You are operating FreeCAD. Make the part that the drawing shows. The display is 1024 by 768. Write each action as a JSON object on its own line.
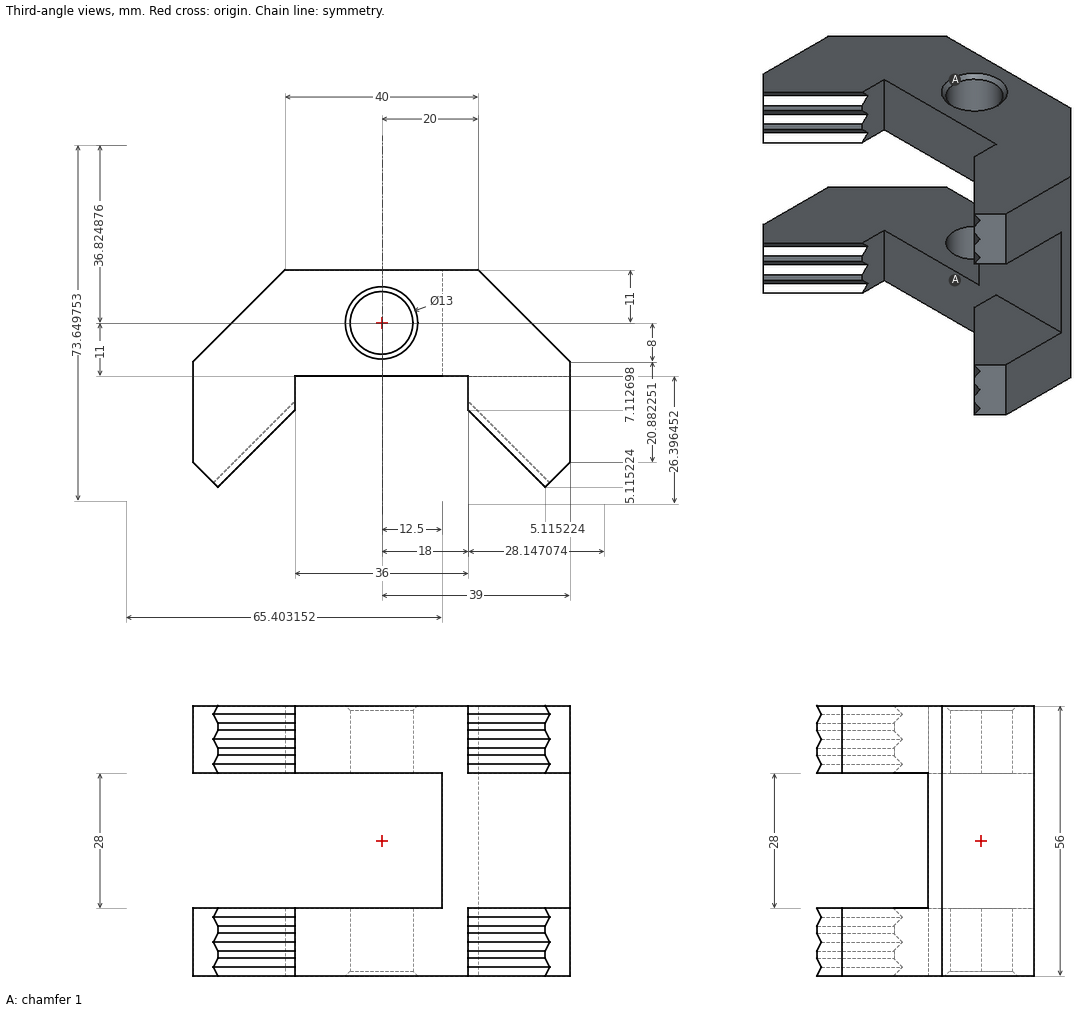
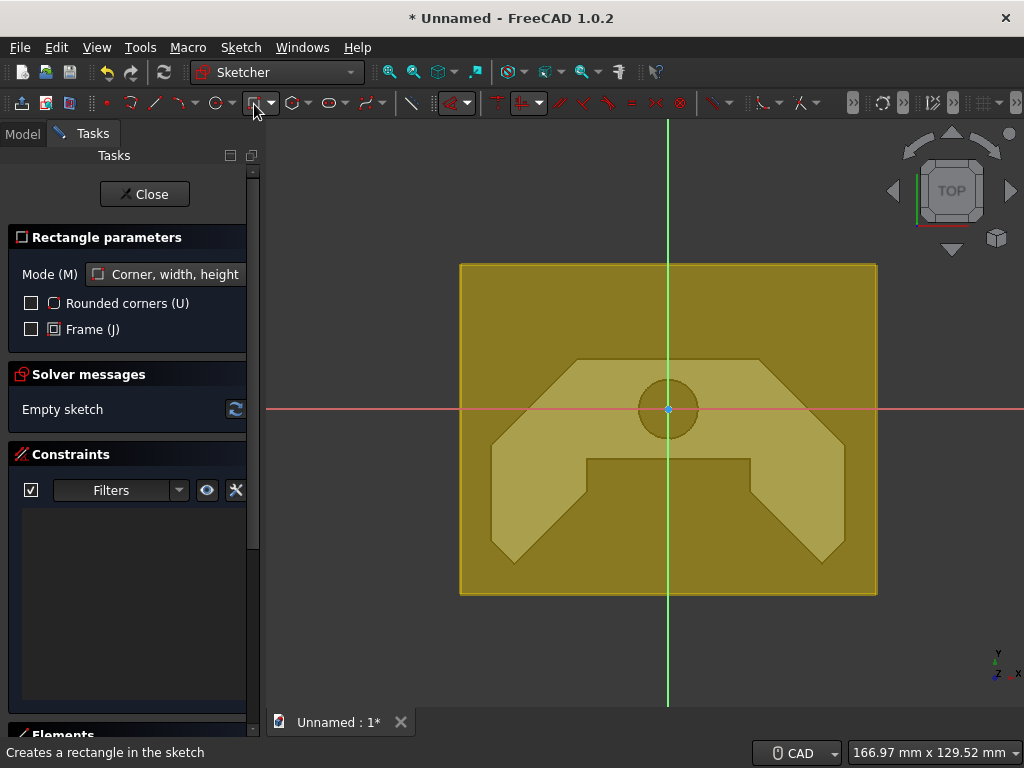
{"action": "left_click", "coordinate": [428, 242]}
{"action": "left_click", "coordinate": [725, 576]}
{"action": "key", "text": "Escape"}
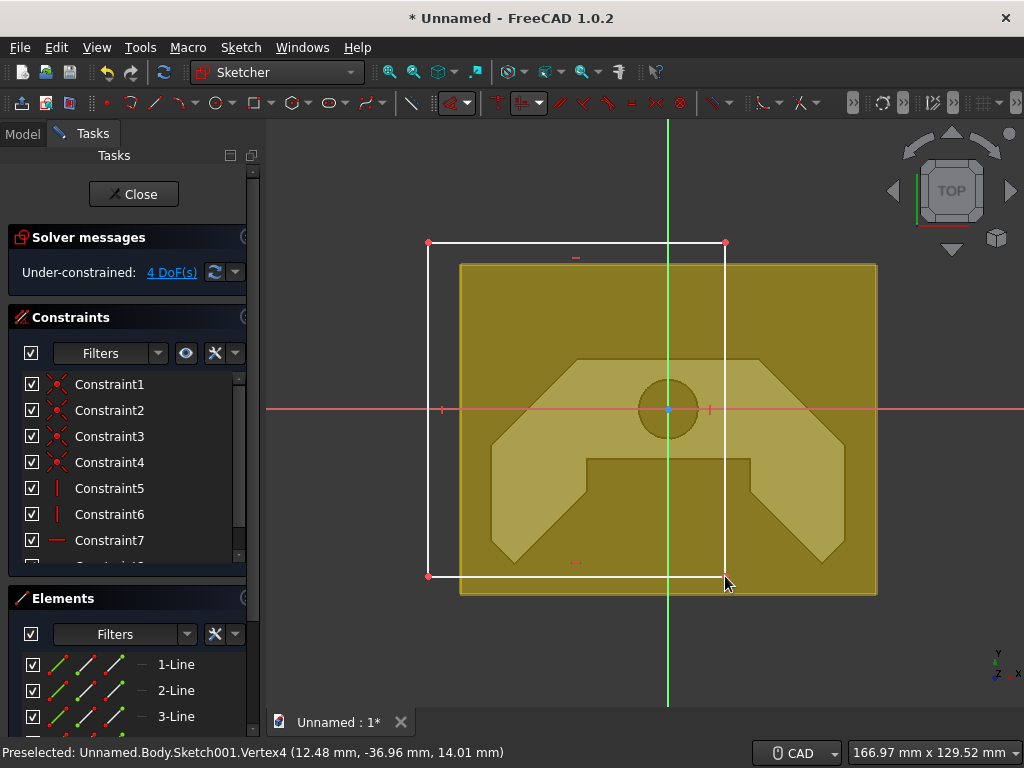
{"action": "left_click", "coordinate": [725, 577]}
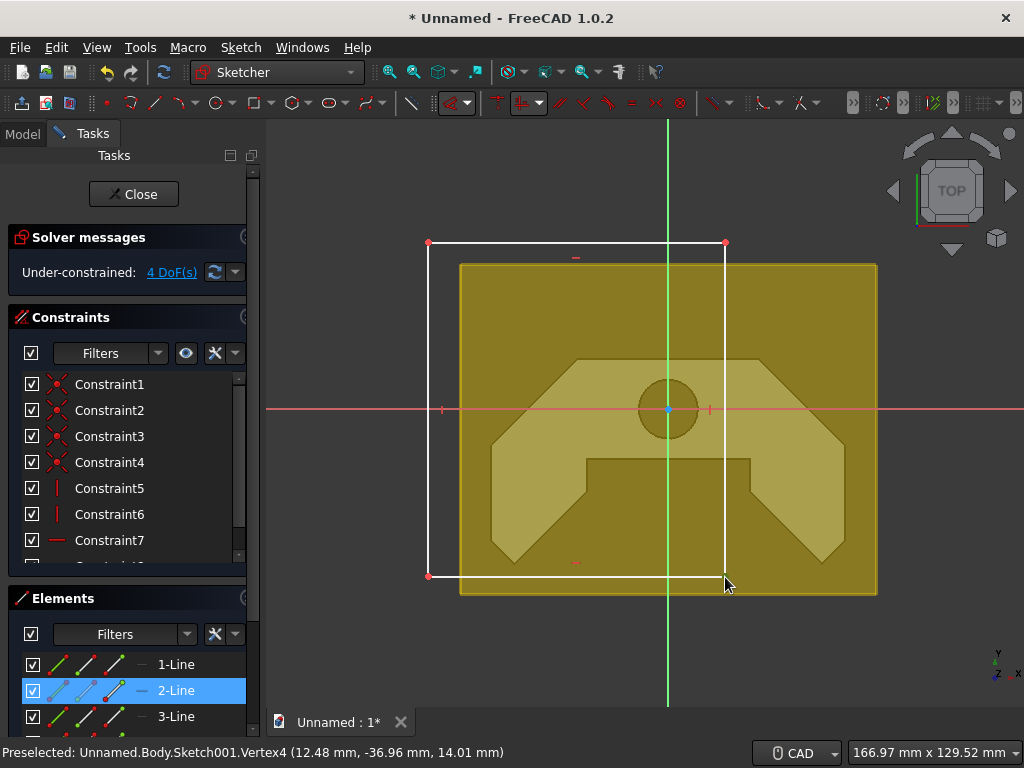
{"action": "left_click", "coordinate": [470, 104]}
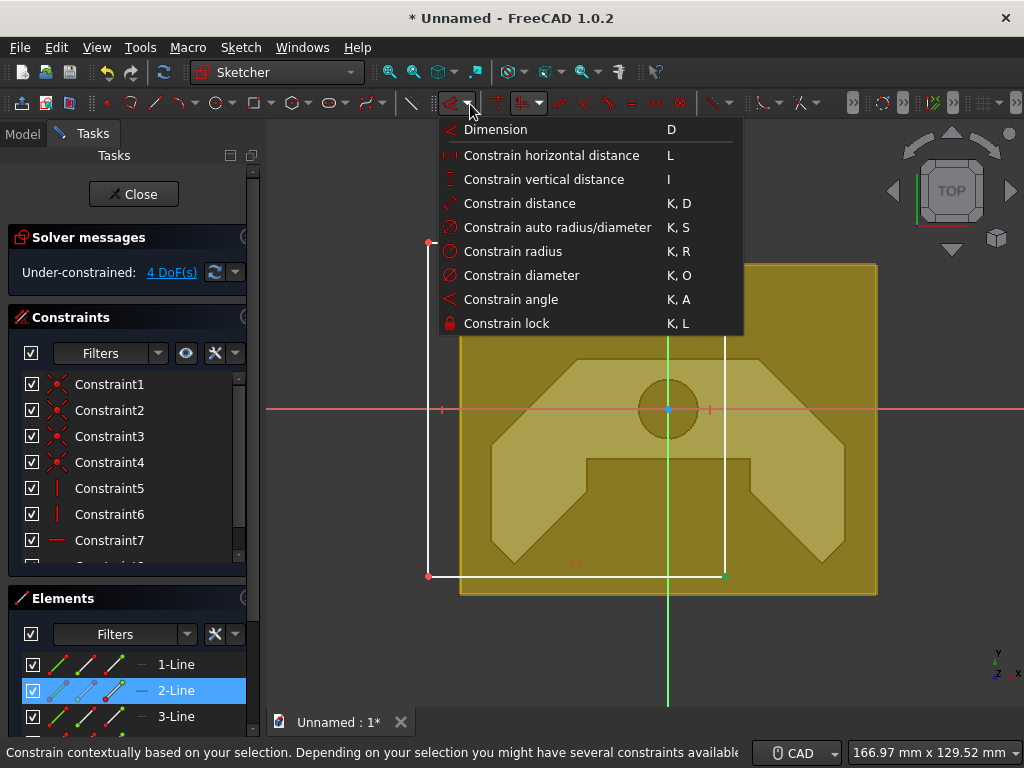
{"action": "left_click", "coordinate": [591, 155]}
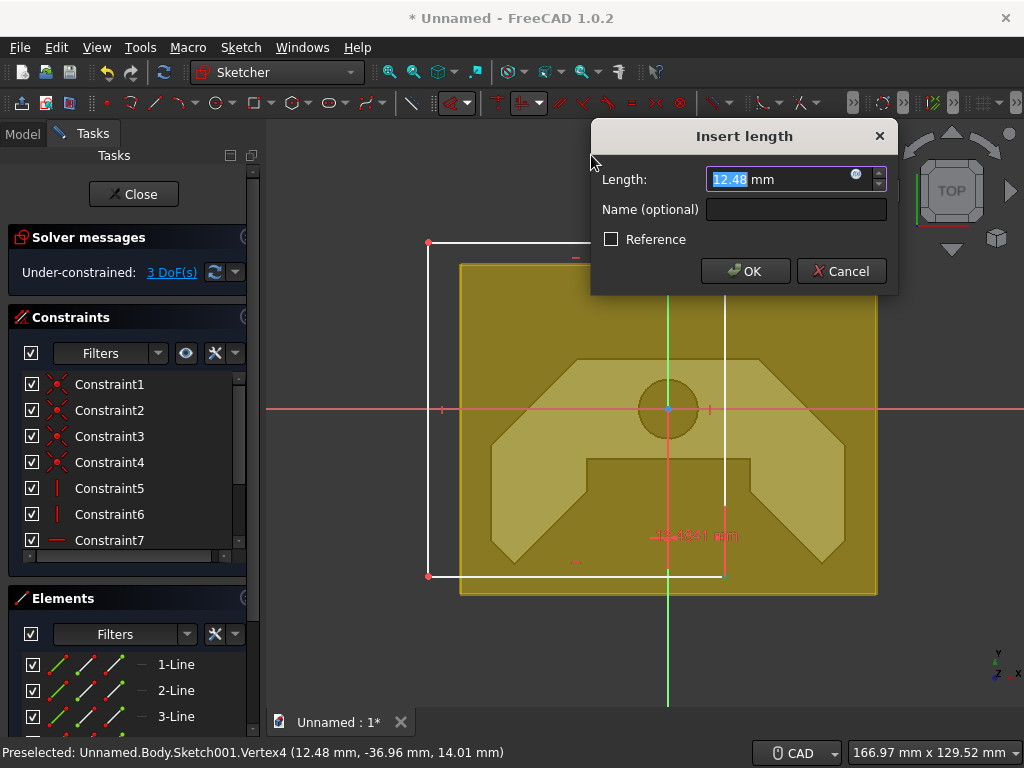
{"action": "type", "text": "12.5"}
{"action": "key", "text": "Return"}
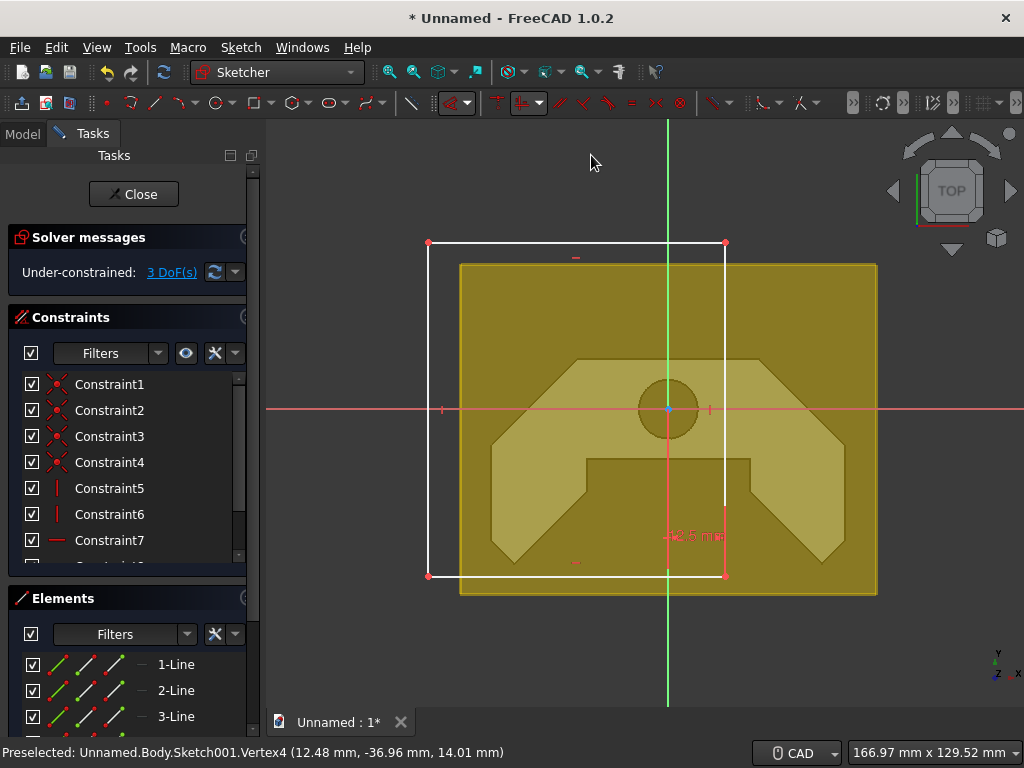
{"action": "left_click", "coordinate": [428, 343]}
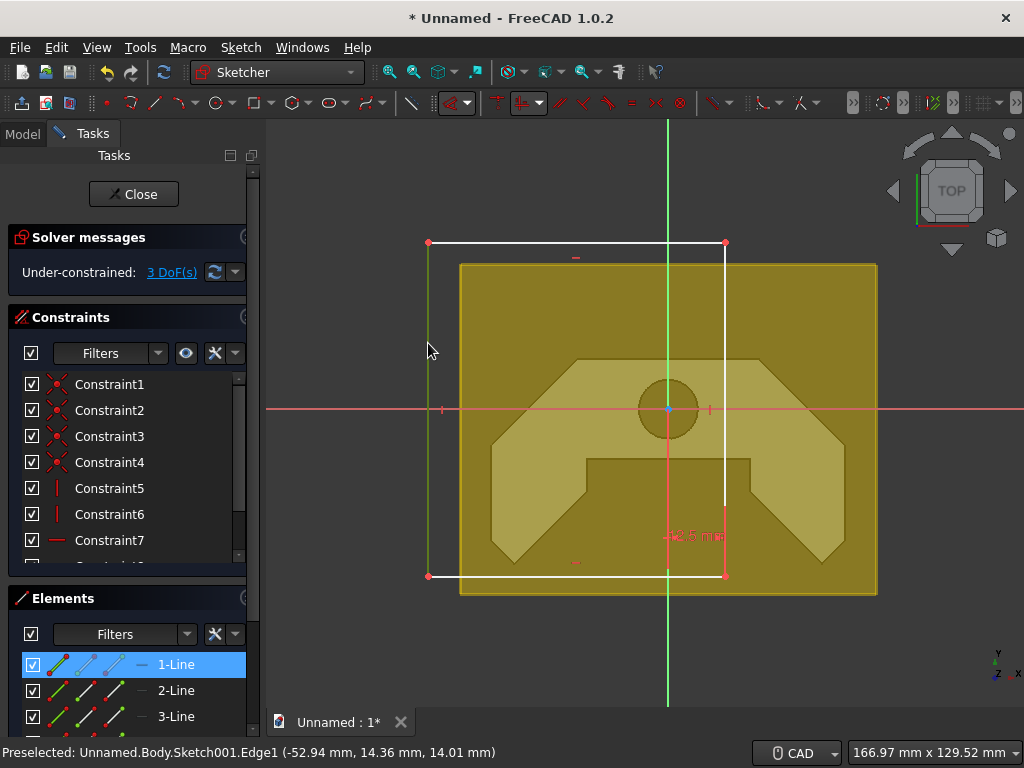
{"action": "key", "text": "i"}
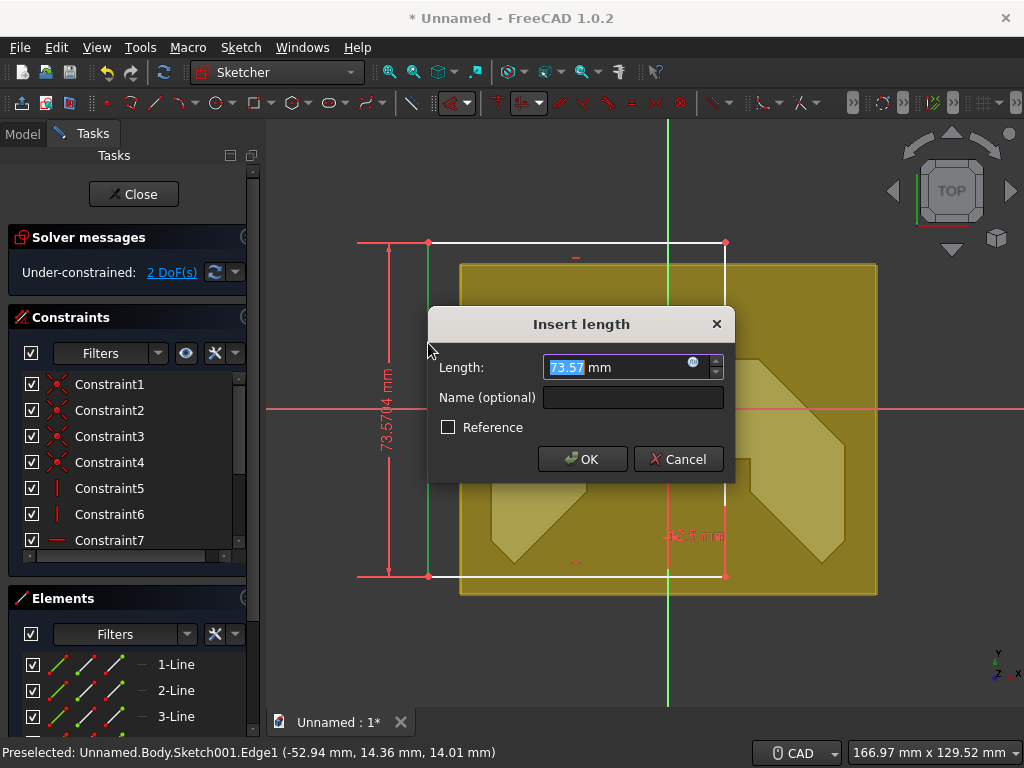
{"action": "type", "text": "73.649753"}
{"action": "key", "text": "Return"}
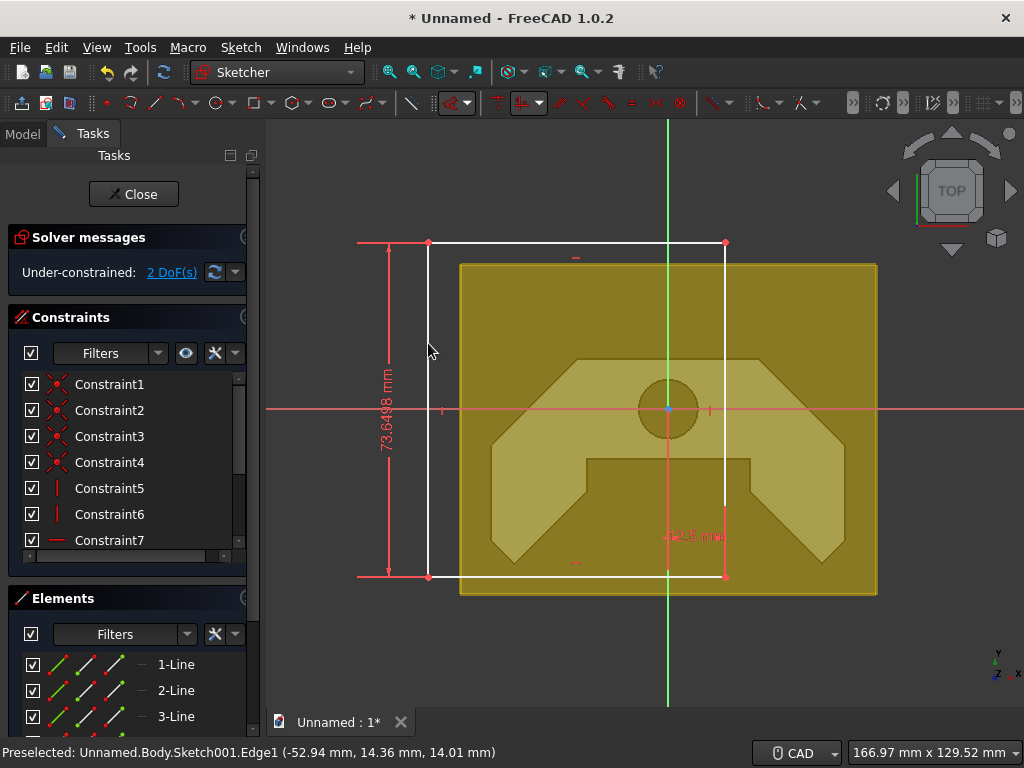
{"action": "left_click", "coordinate": [517, 577]}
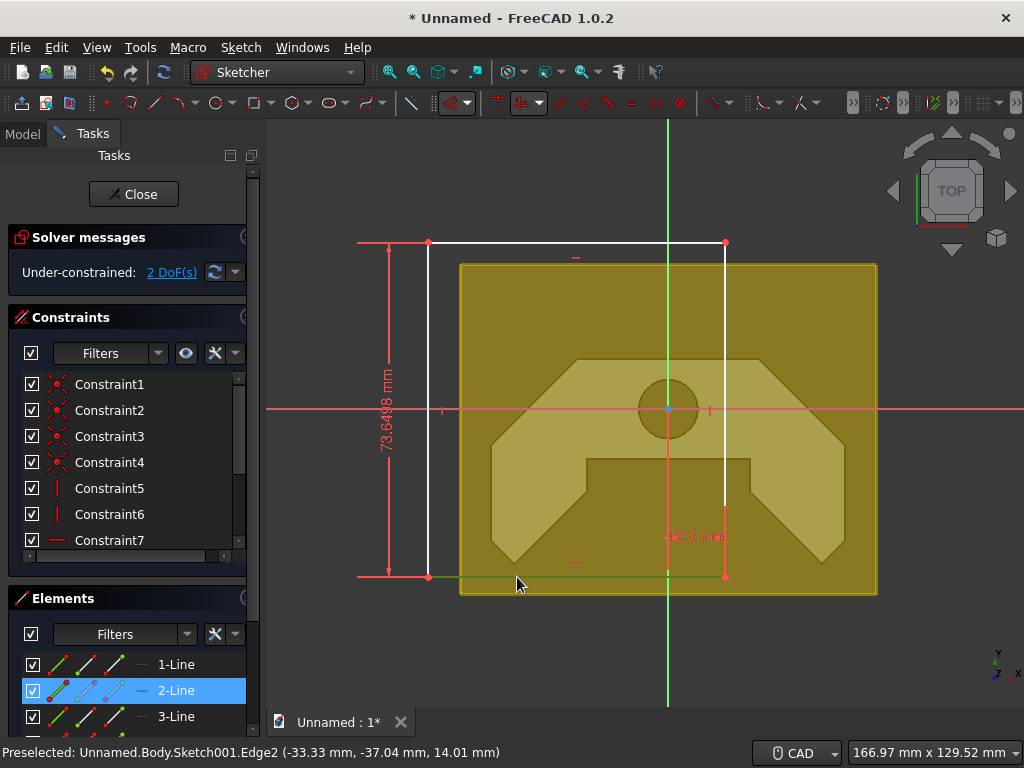
{"action": "key", "text": "l"}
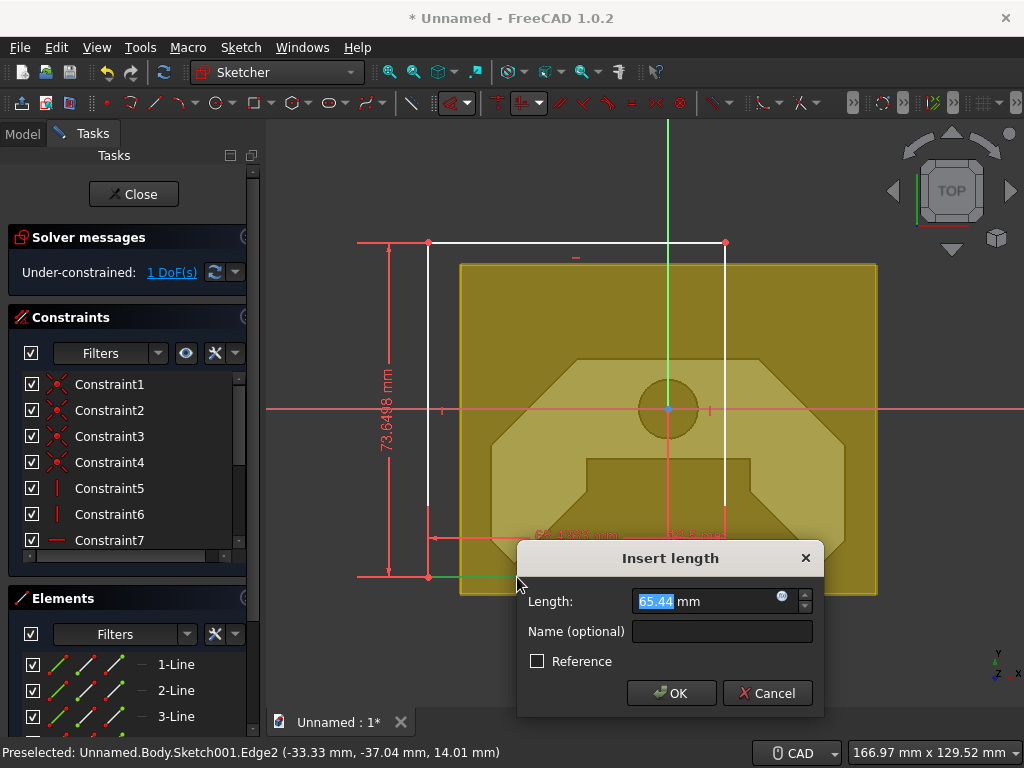
{"action": "type", "text": "65.403152"}
{"action": "key", "text": "Return"}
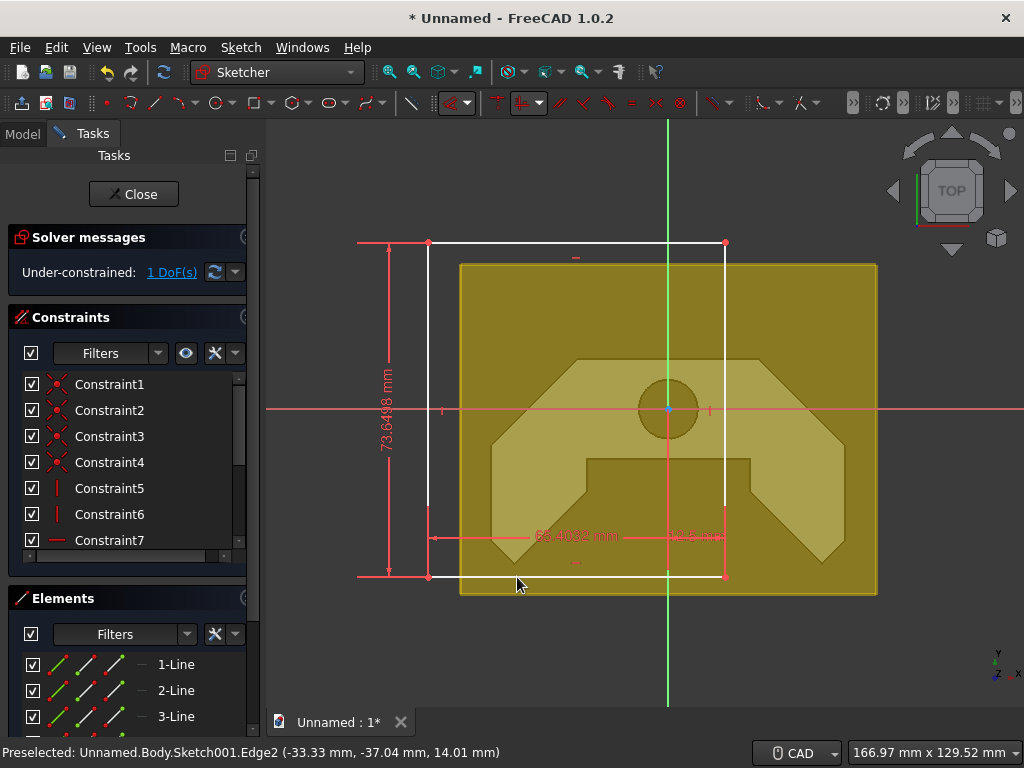
{"action": "left_click", "coordinate": [428, 243]}